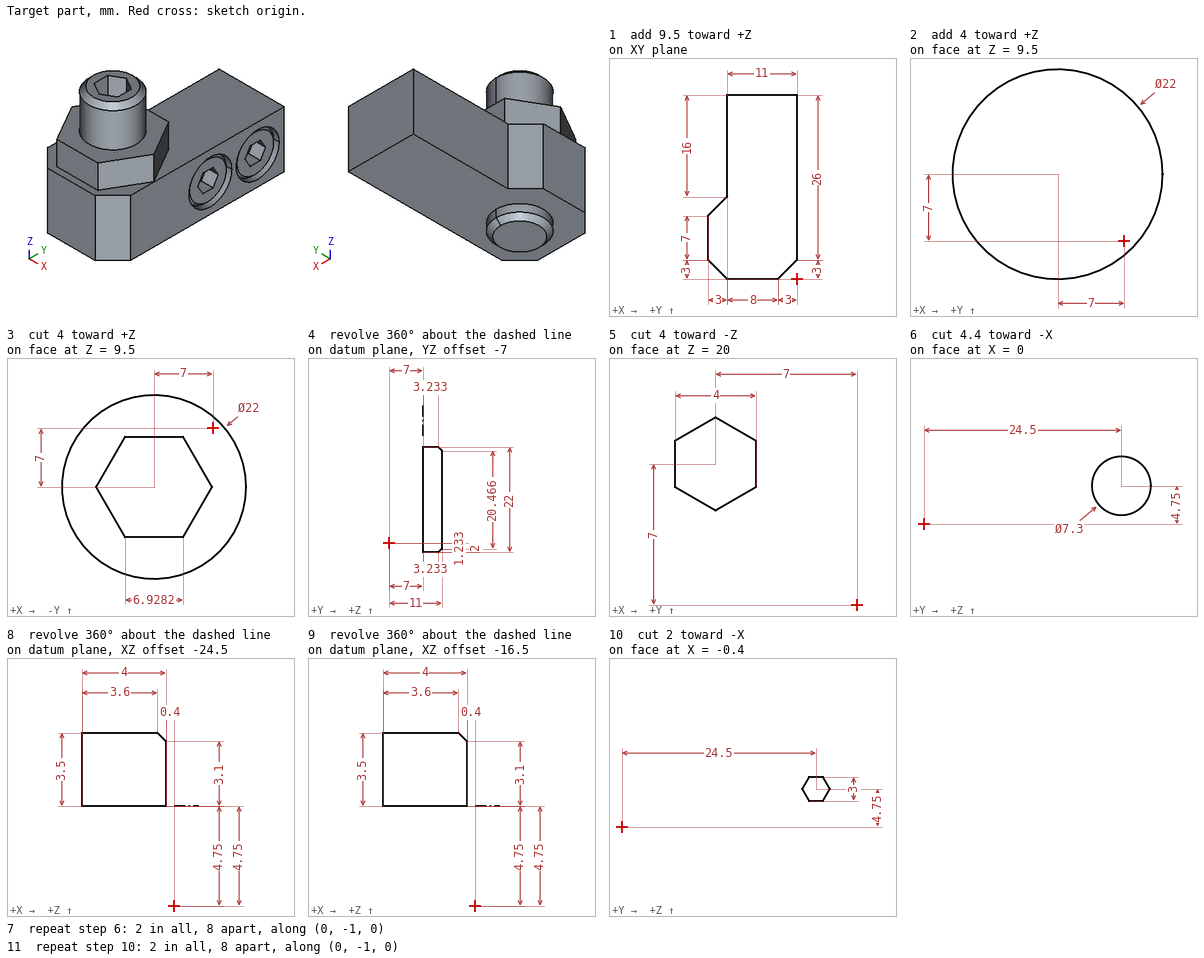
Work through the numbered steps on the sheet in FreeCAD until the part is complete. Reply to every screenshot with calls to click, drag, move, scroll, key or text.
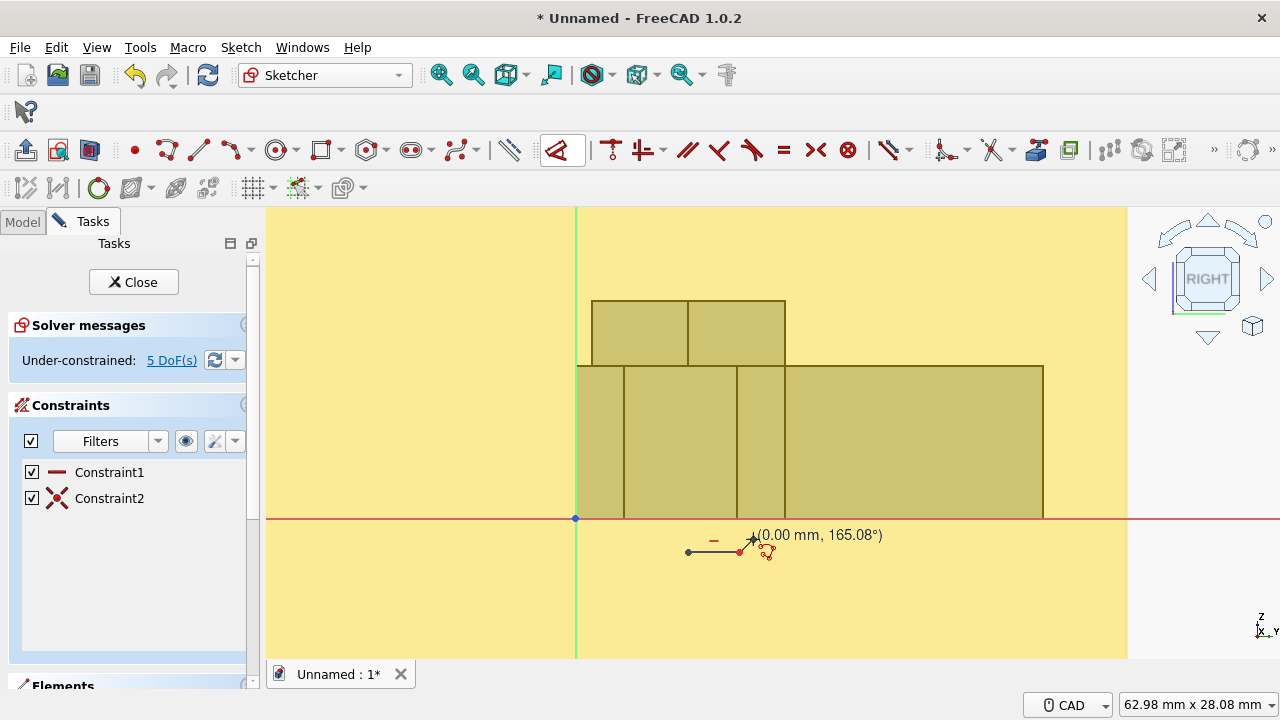
scroll(753, 591, down, 3)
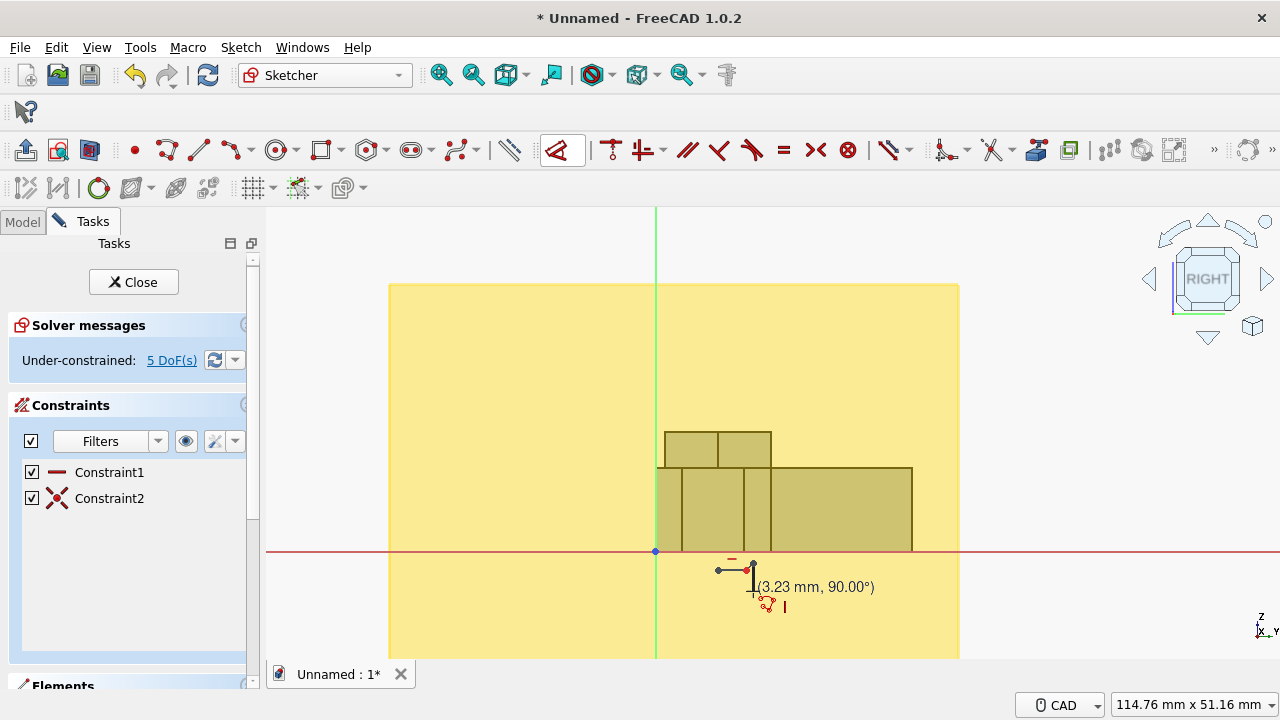
click(753, 382)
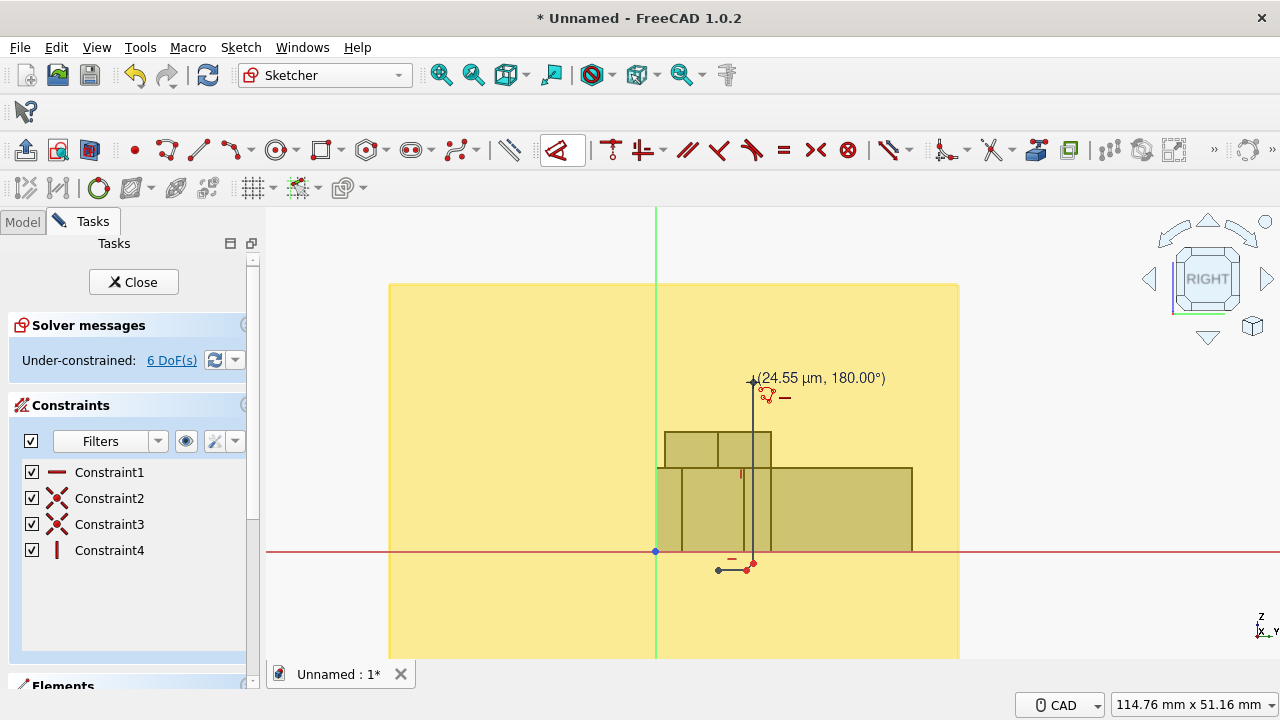
scroll(746, 375, up, 3)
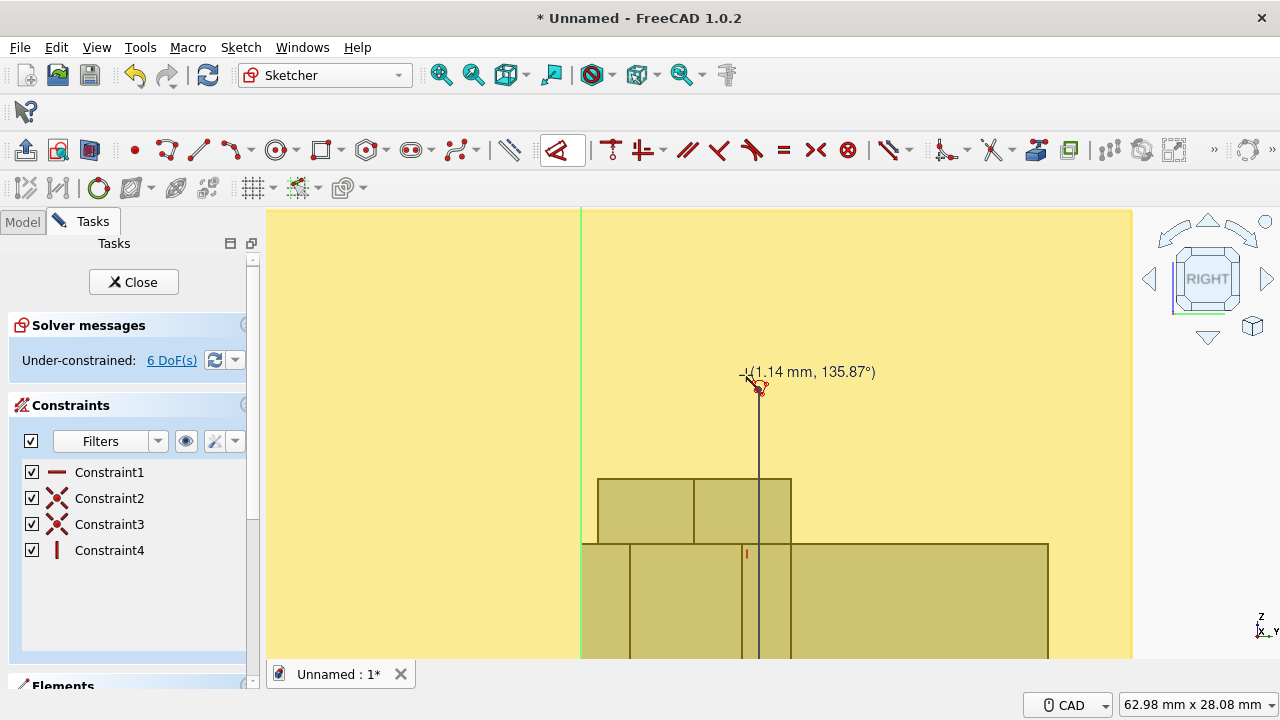
click(746, 375)
click(694, 375)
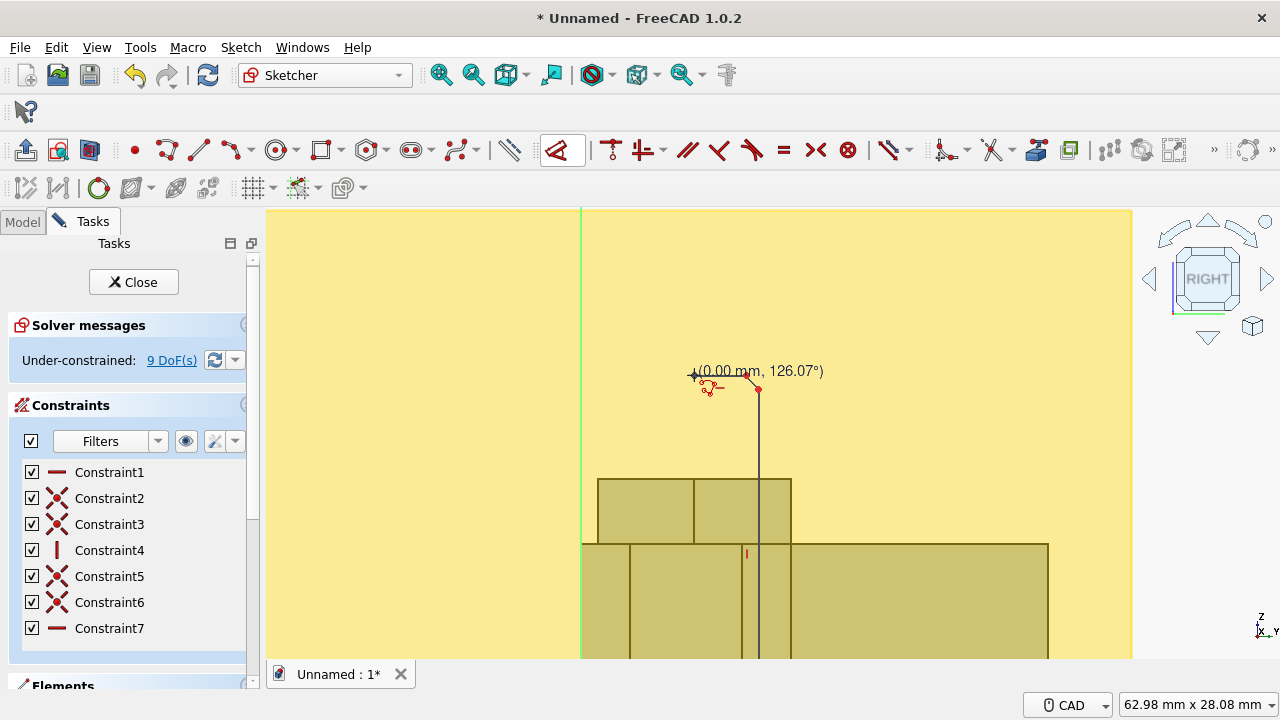
scroll(746, 375, down, 3)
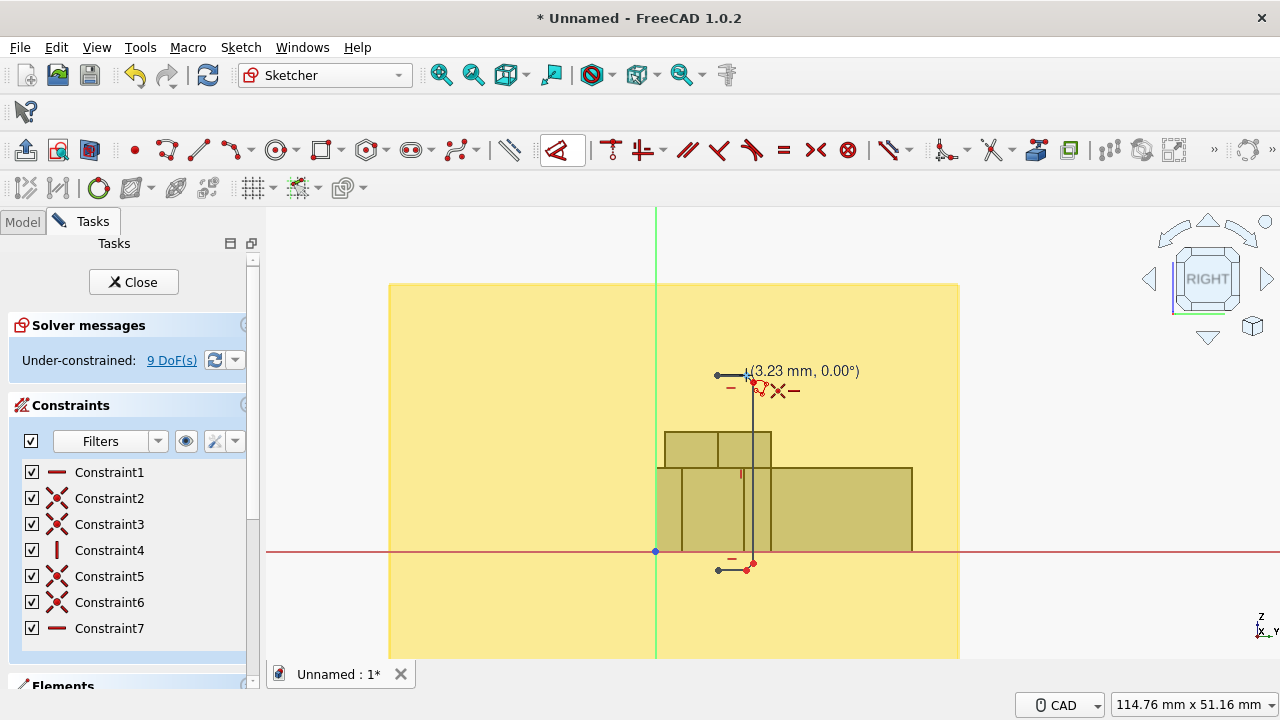
click(718, 570)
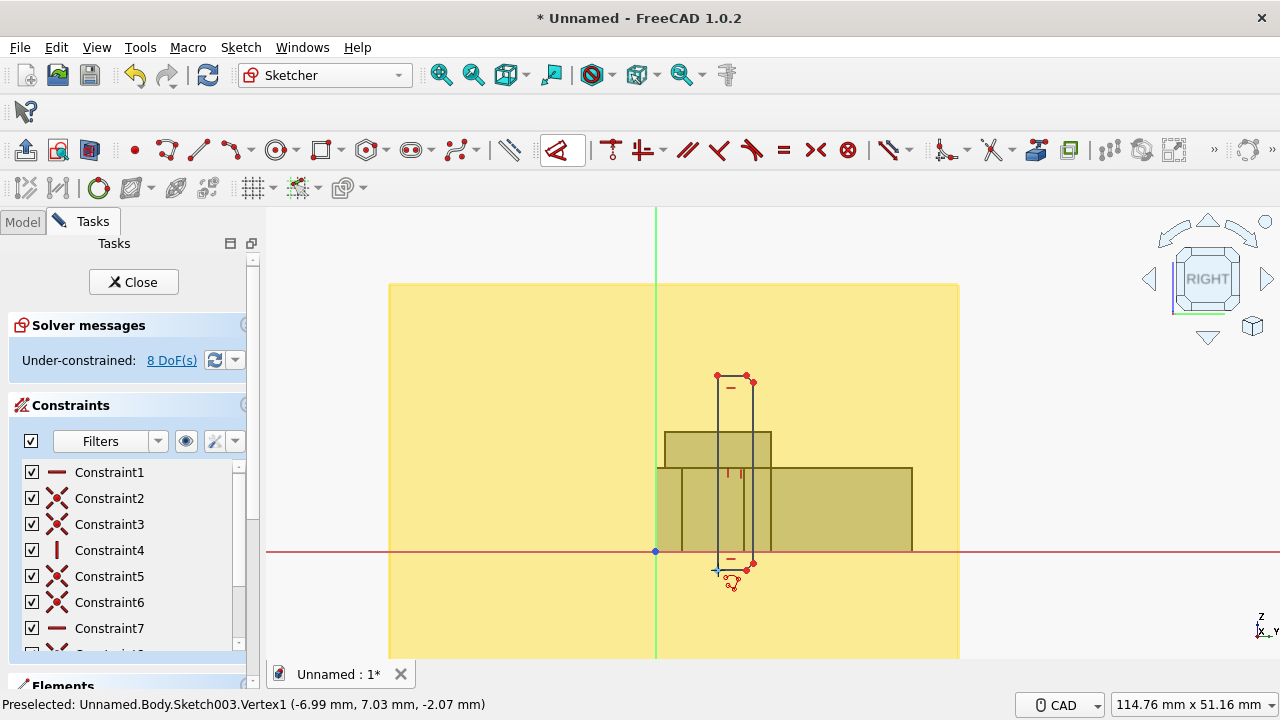
key(g)
key(l)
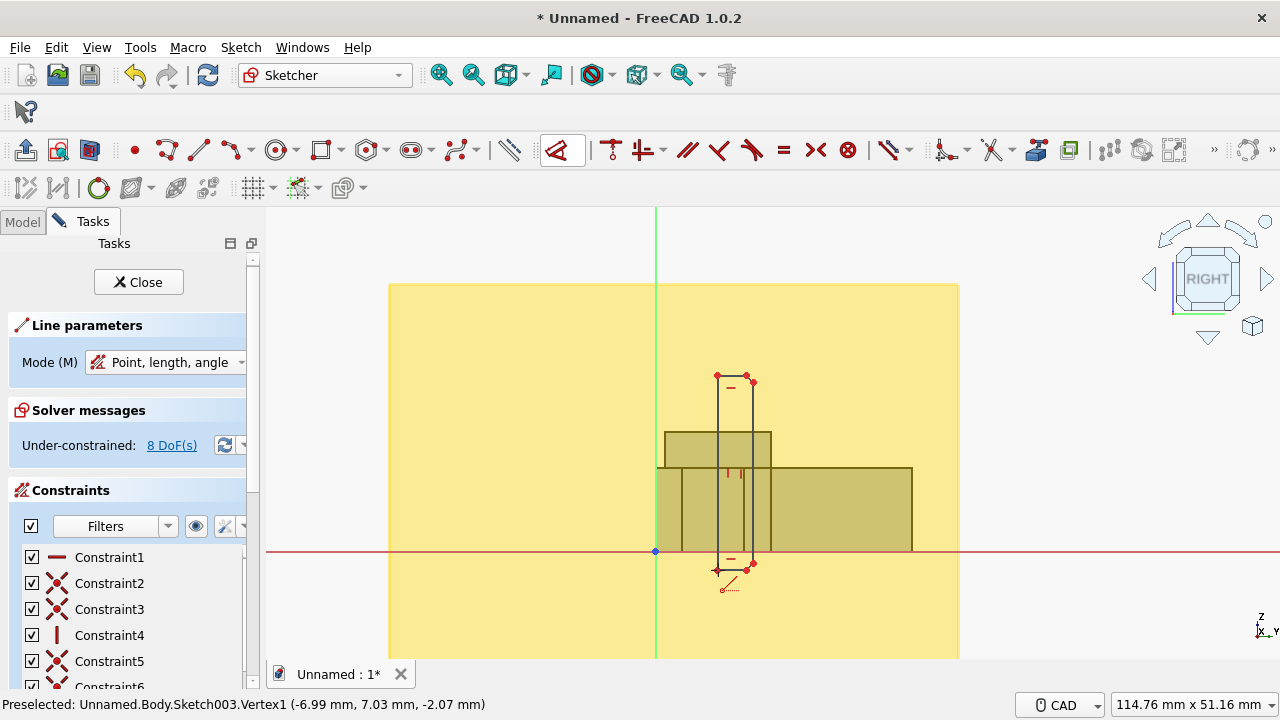
click(718, 356)
click(718, 297)
key(Escape)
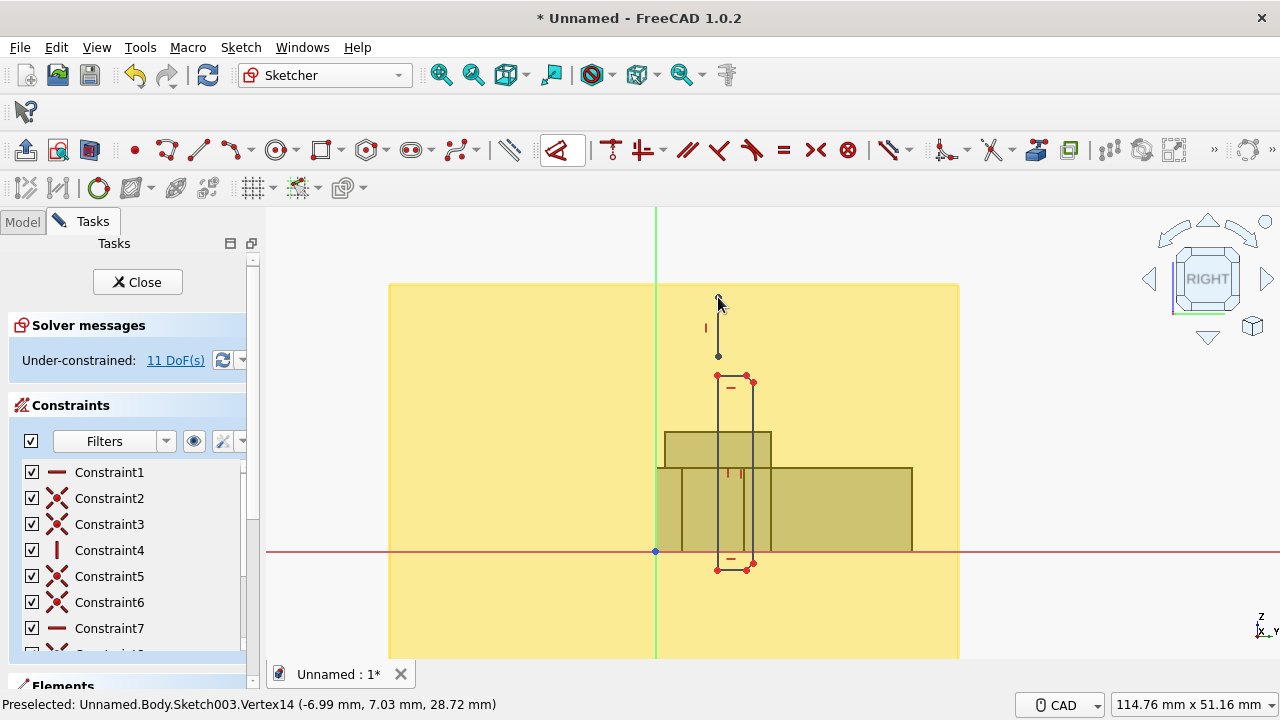
click(718, 339)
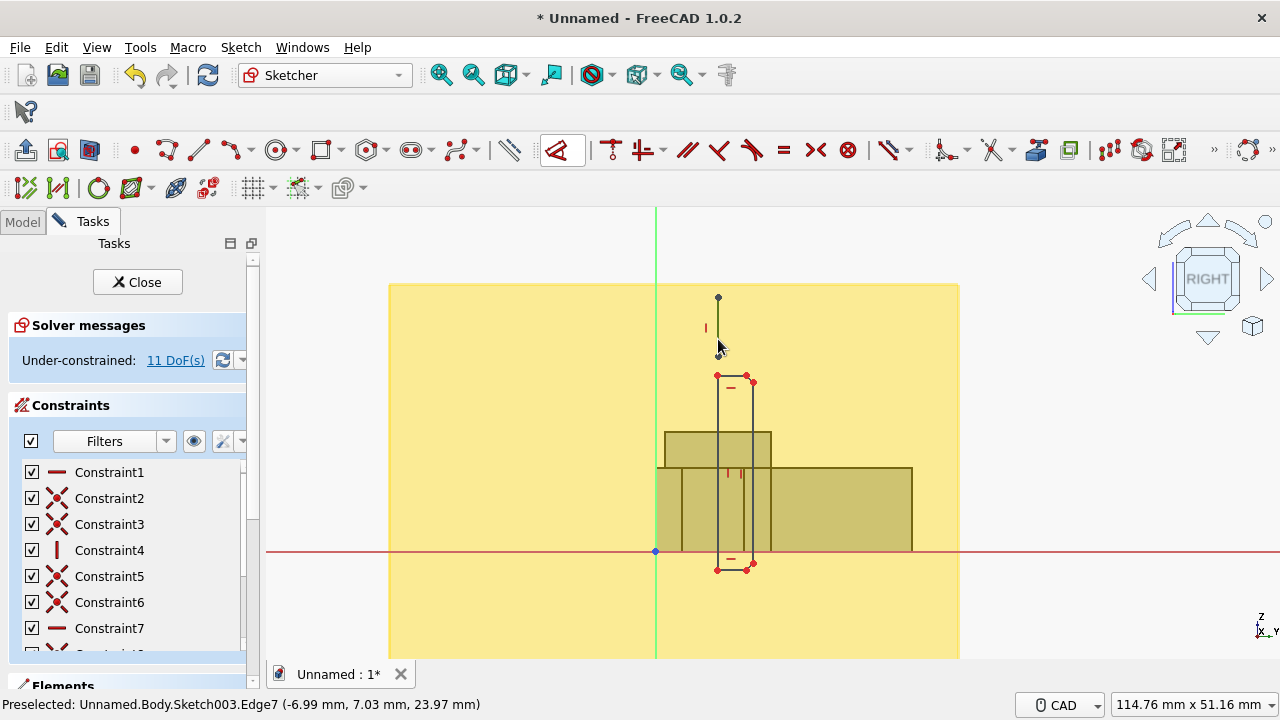
click(510, 150)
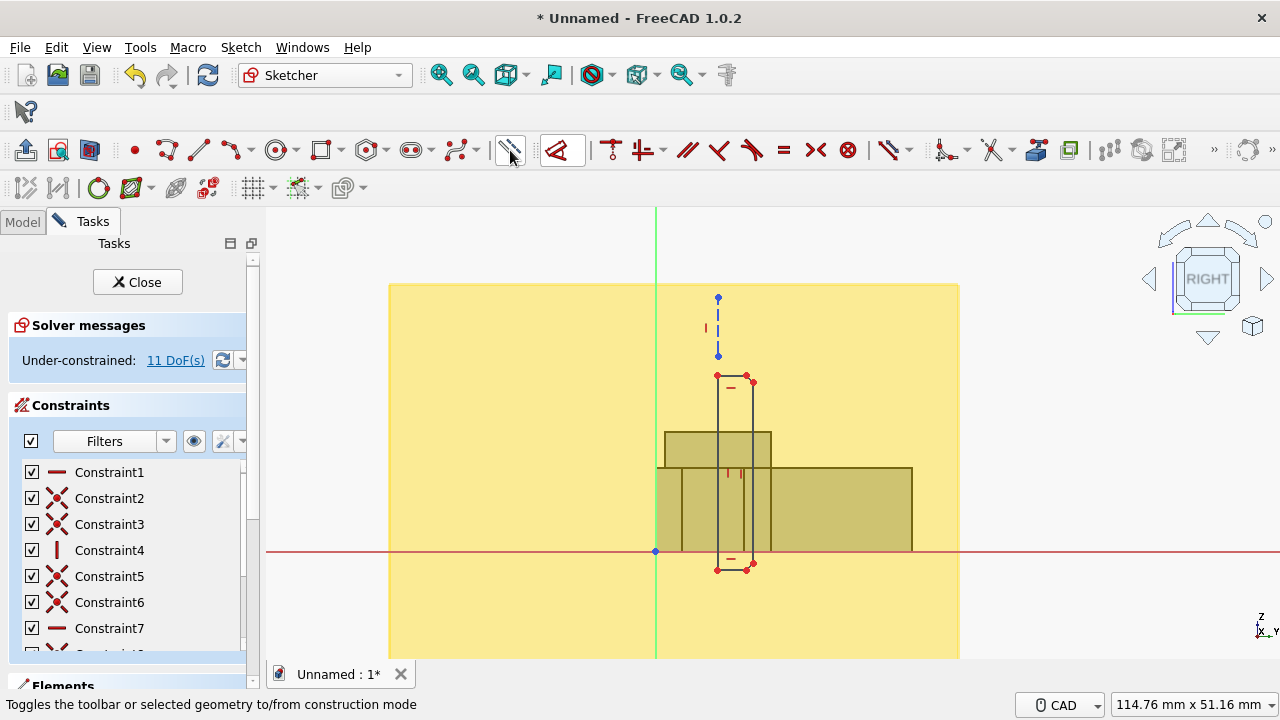
click(718, 434)